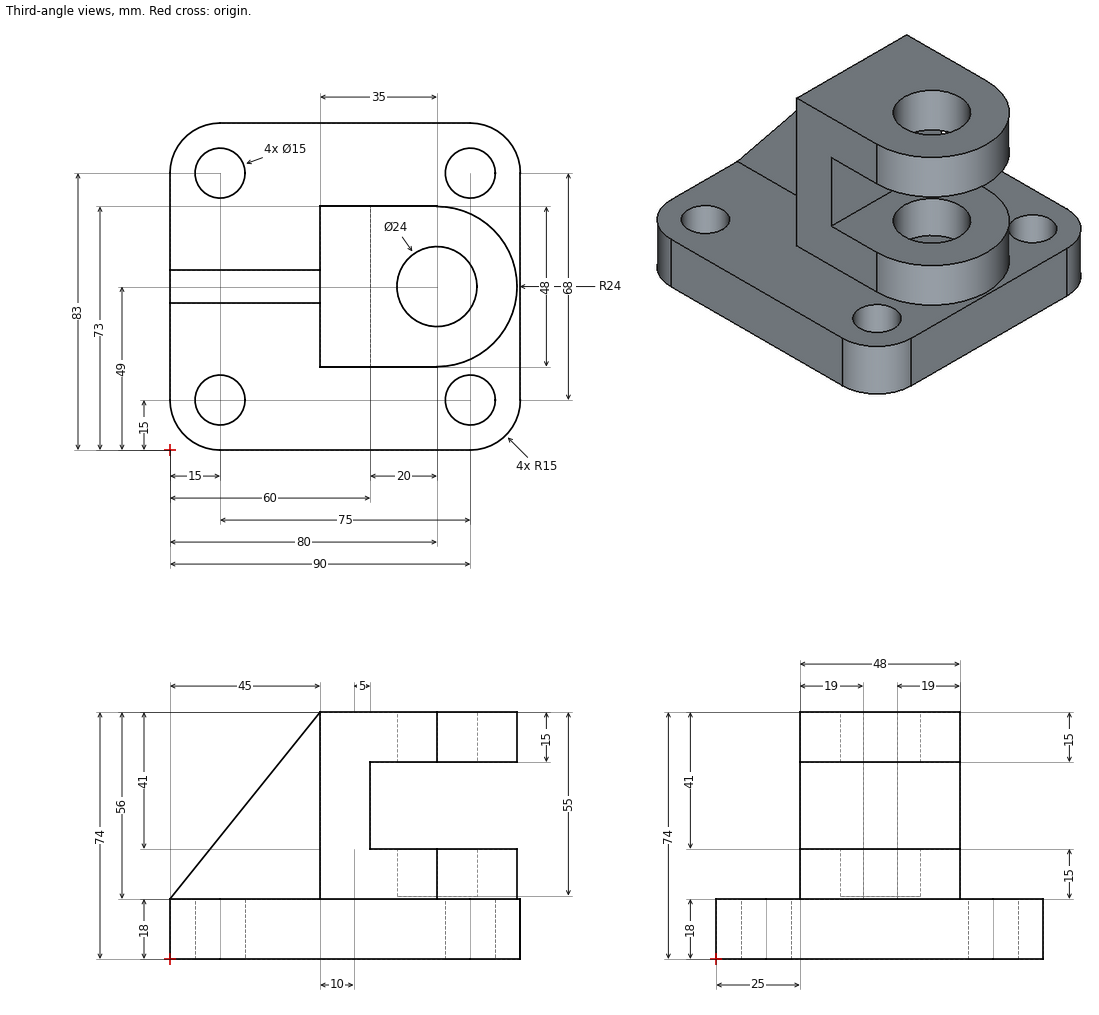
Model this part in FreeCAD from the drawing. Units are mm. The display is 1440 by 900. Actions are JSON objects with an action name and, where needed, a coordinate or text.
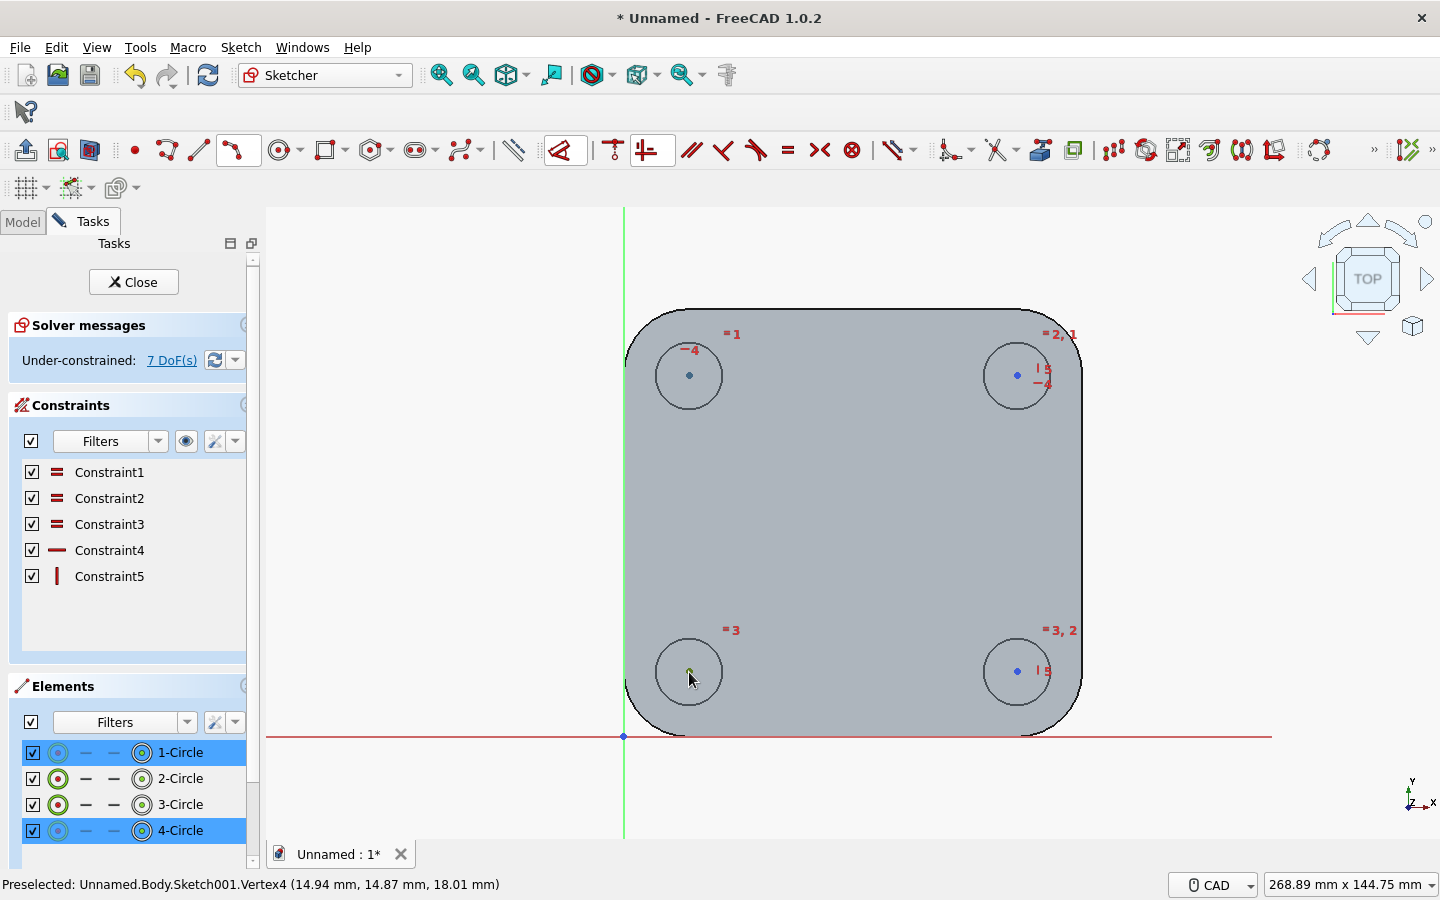
{"action": "left_click", "coordinate": [670, 150]}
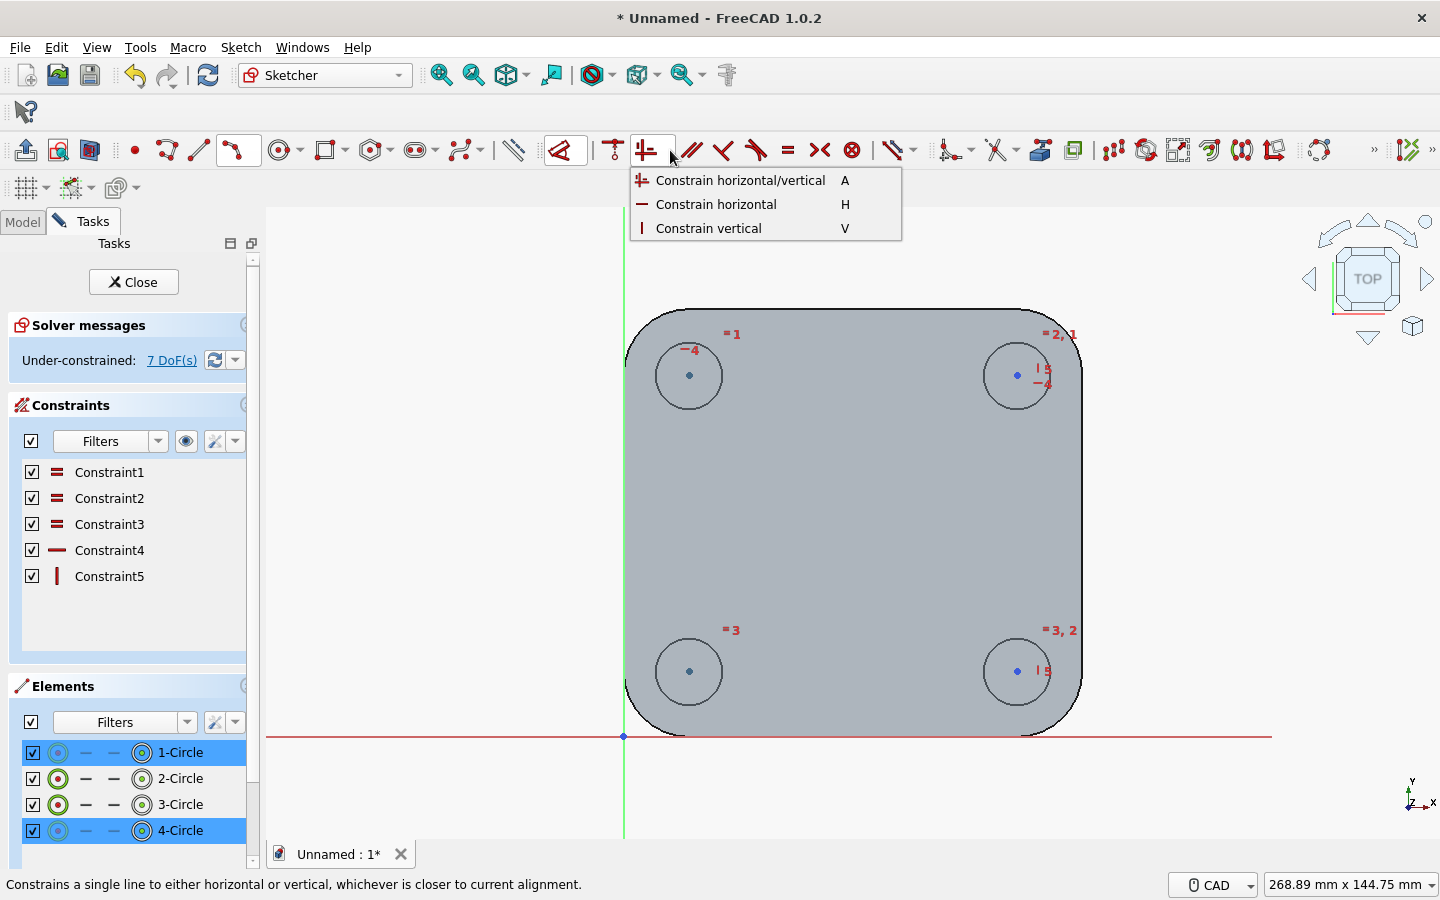
{"action": "left_click", "coordinate": [766, 228]}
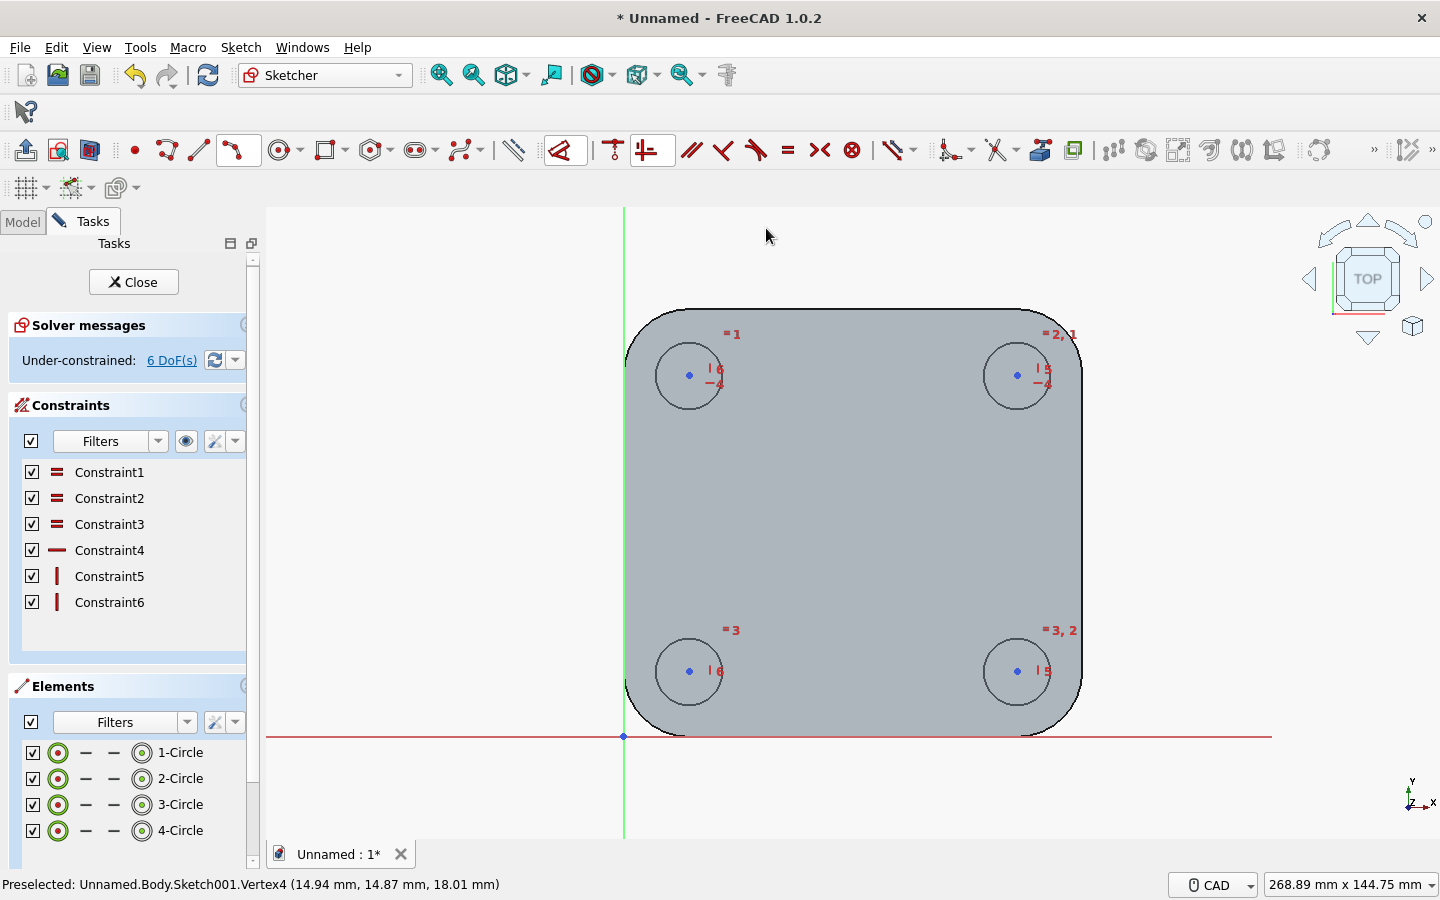
{"action": "left_click", "coordinate": [1017, 672]}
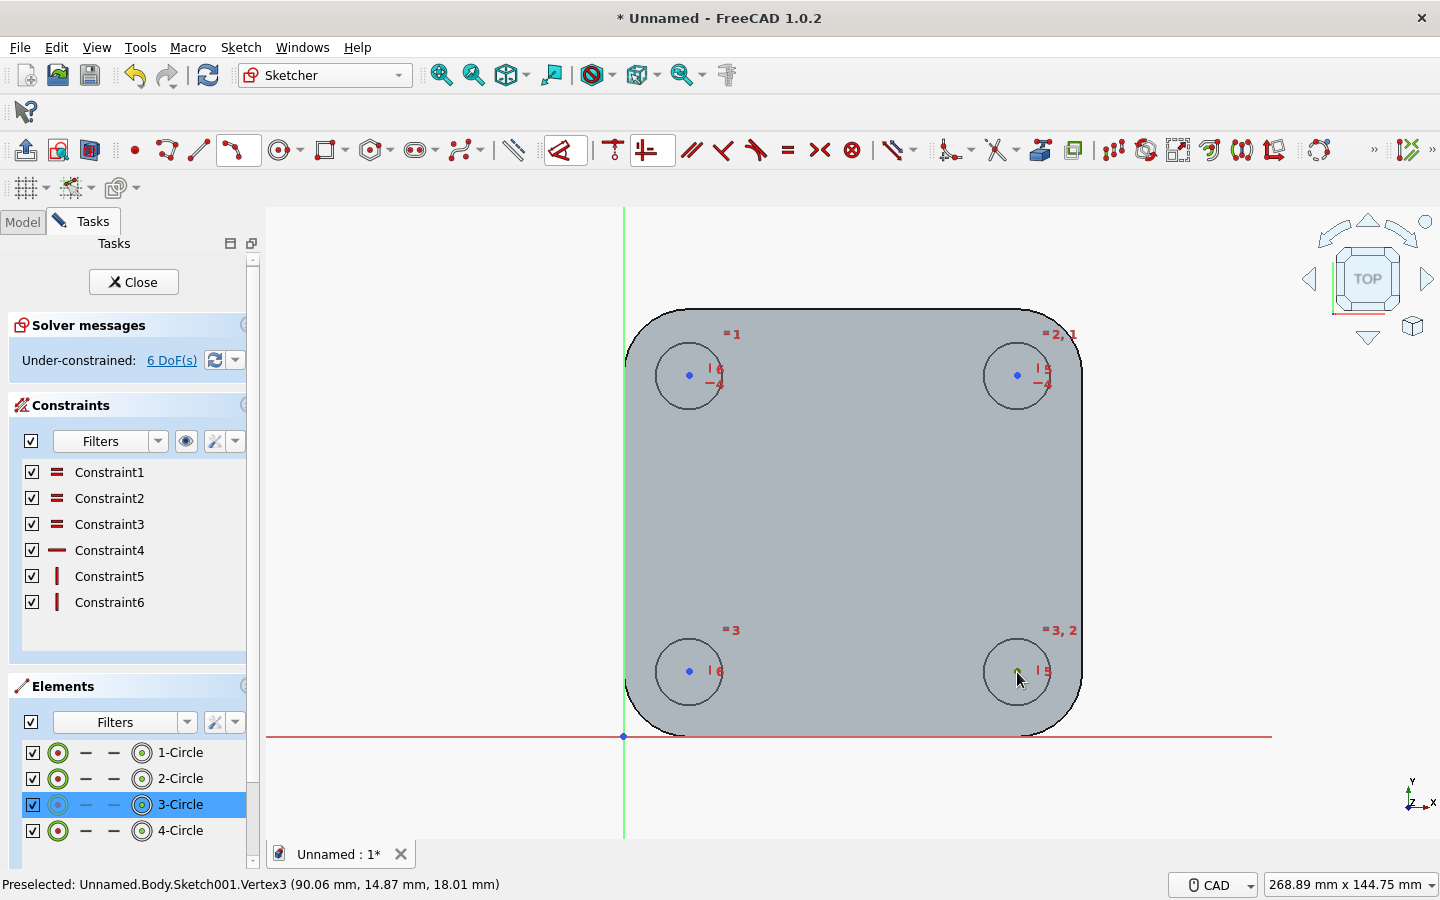
{"action": "left_click", "coordinate": [689, 672]}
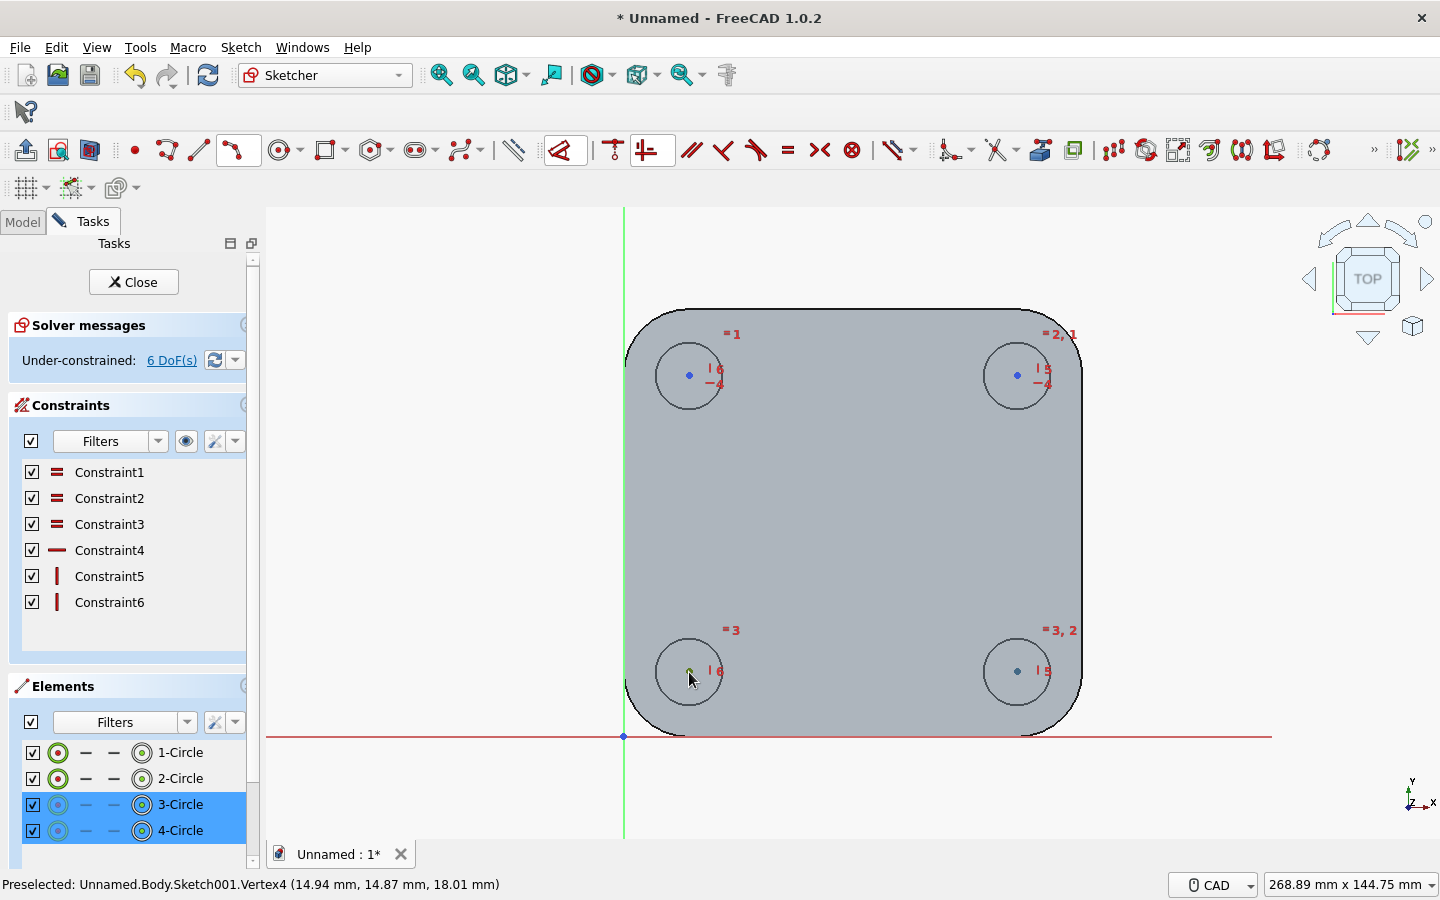
{"action": "key", "text": "h"}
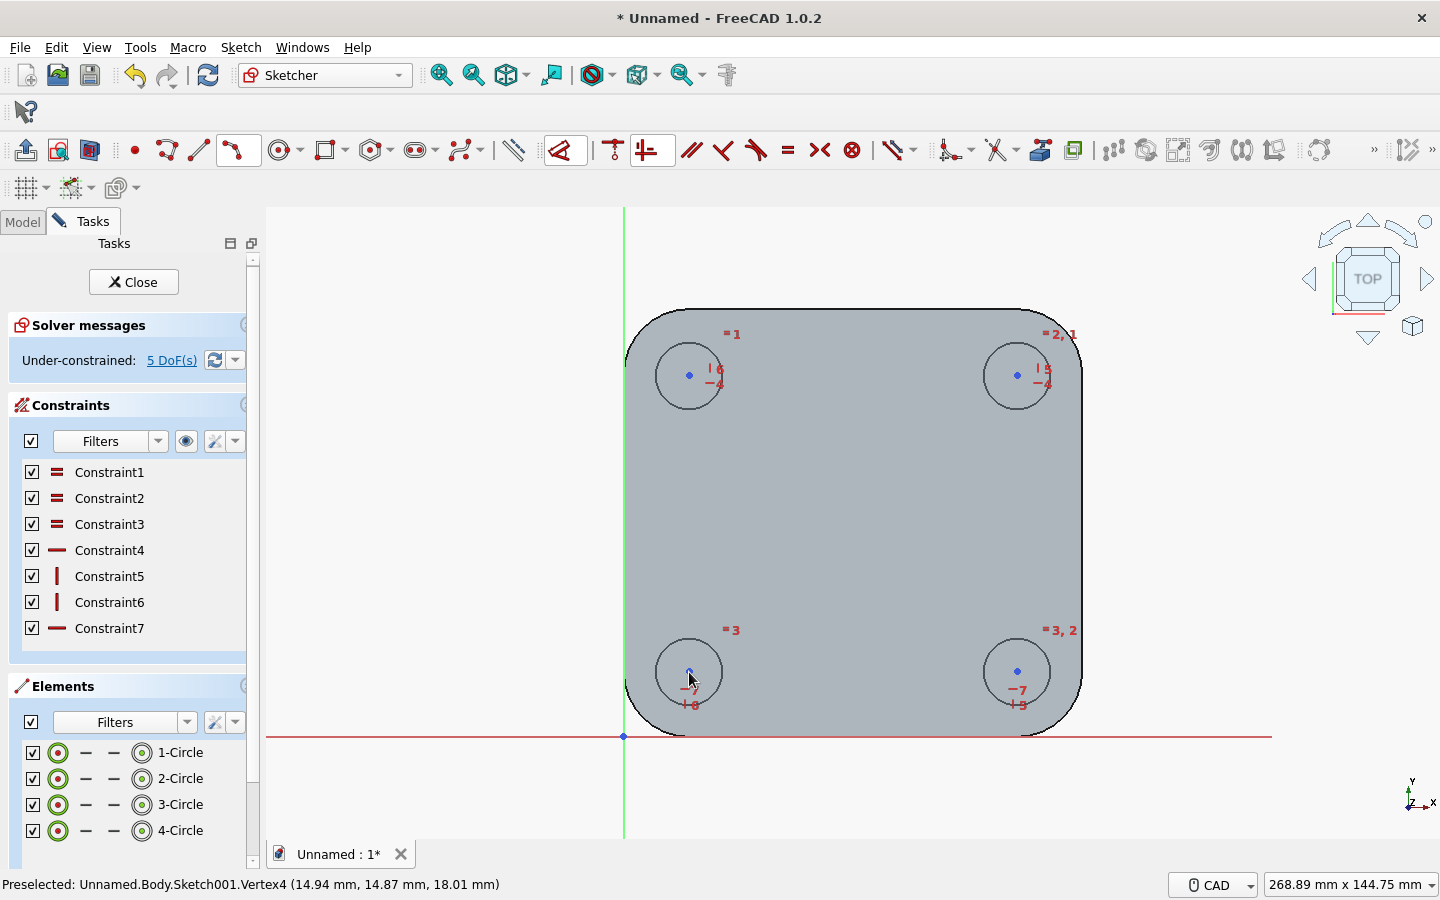
{"action": "left_click", "coordinate": [712, 352]}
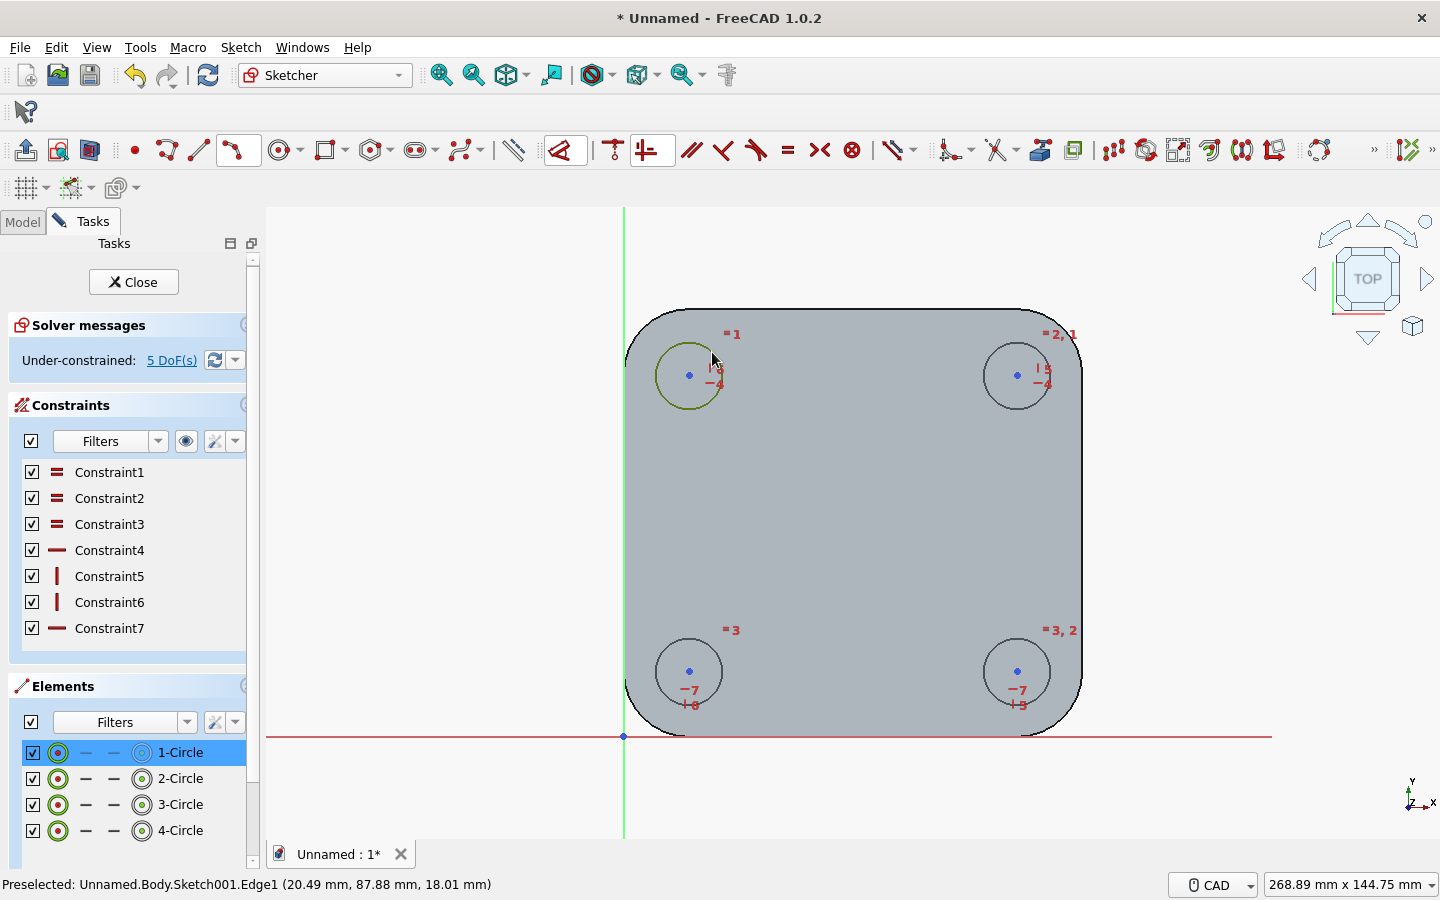
{"action": "key", "text": "k o"}